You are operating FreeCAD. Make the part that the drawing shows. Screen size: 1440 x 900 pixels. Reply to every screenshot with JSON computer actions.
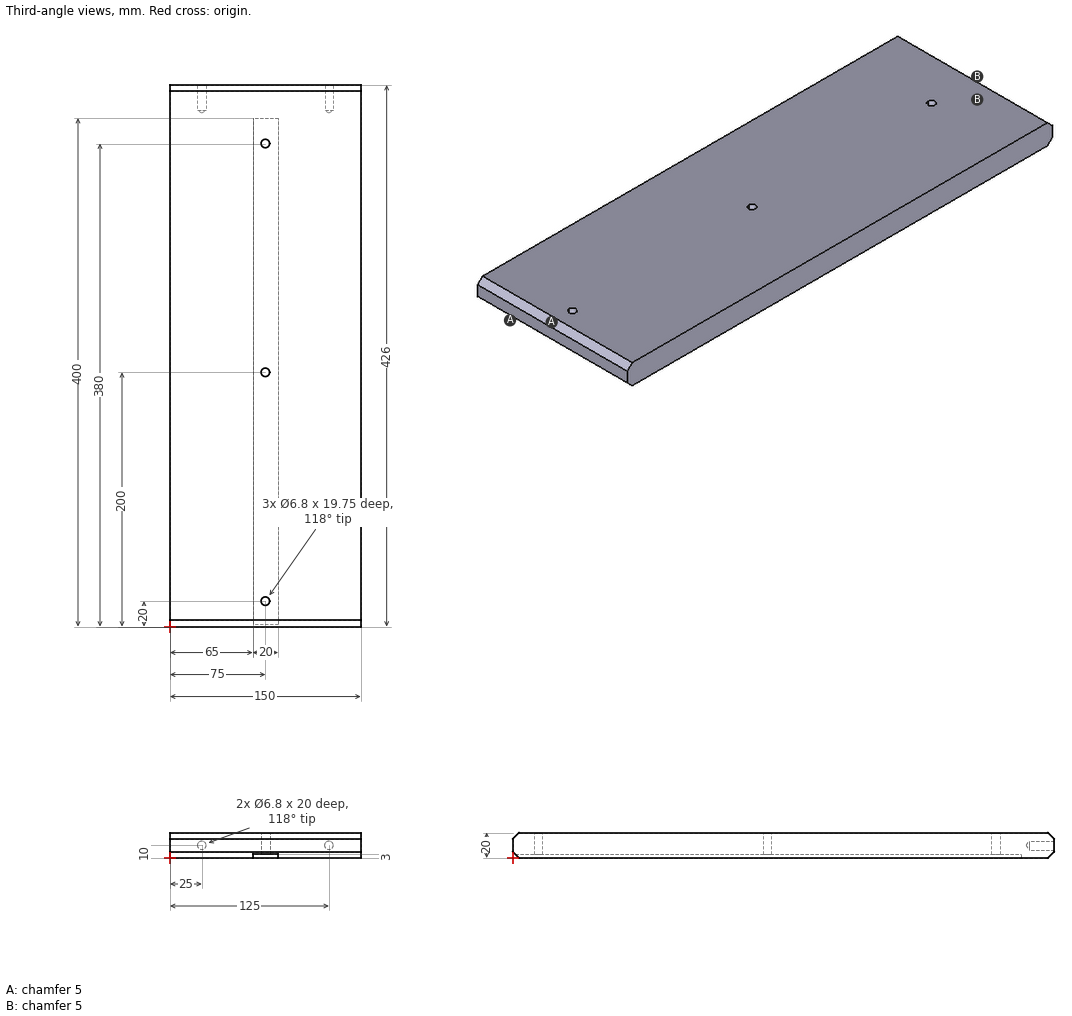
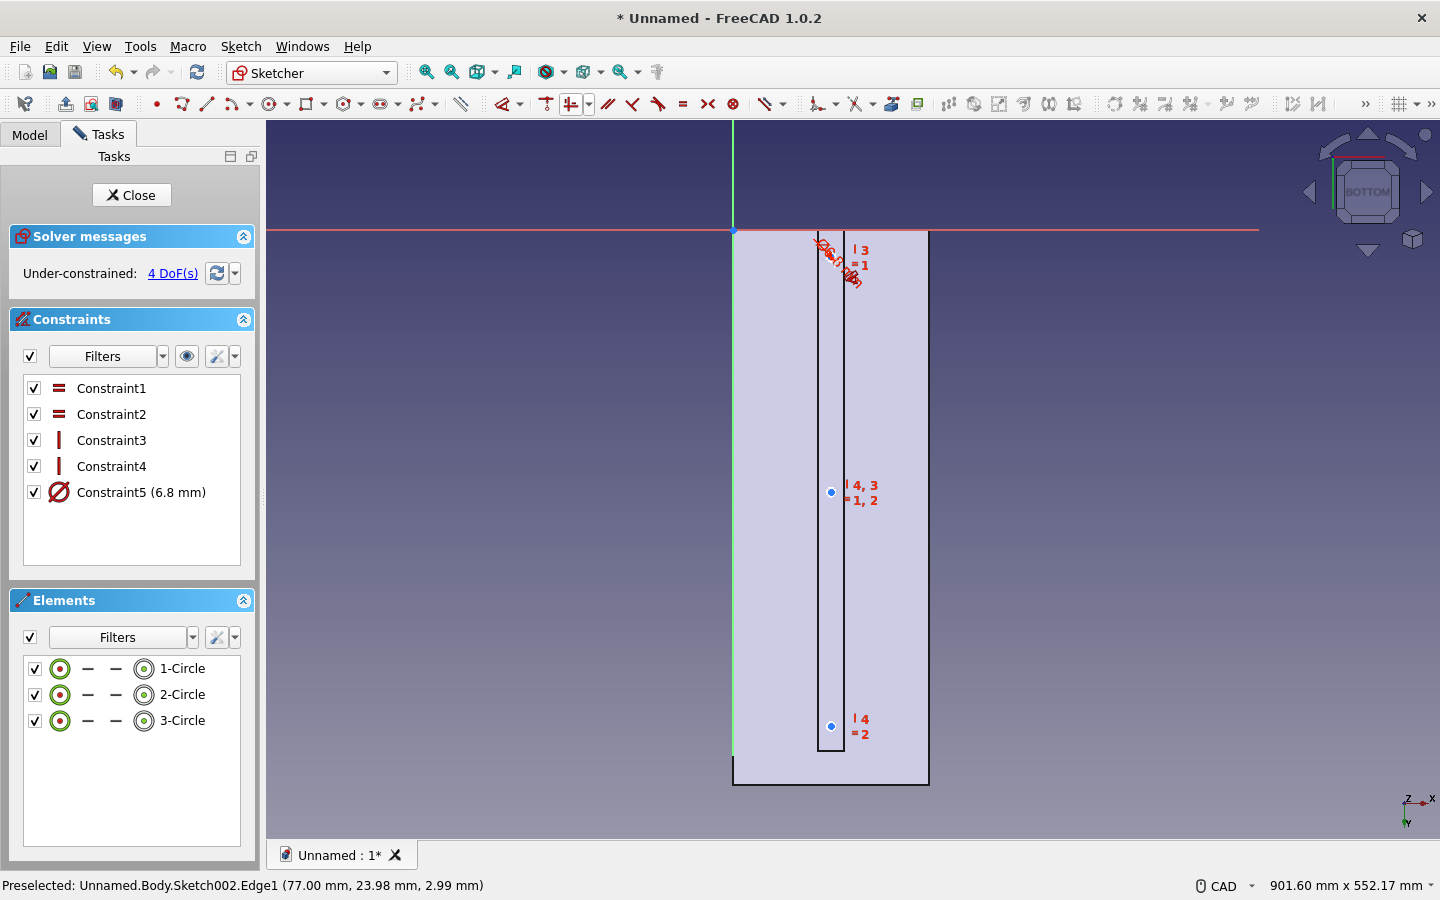
{"action": "left_click", "coordinate": [831, 257]}
{"action": "left_click", "coordinate": [782, 196]}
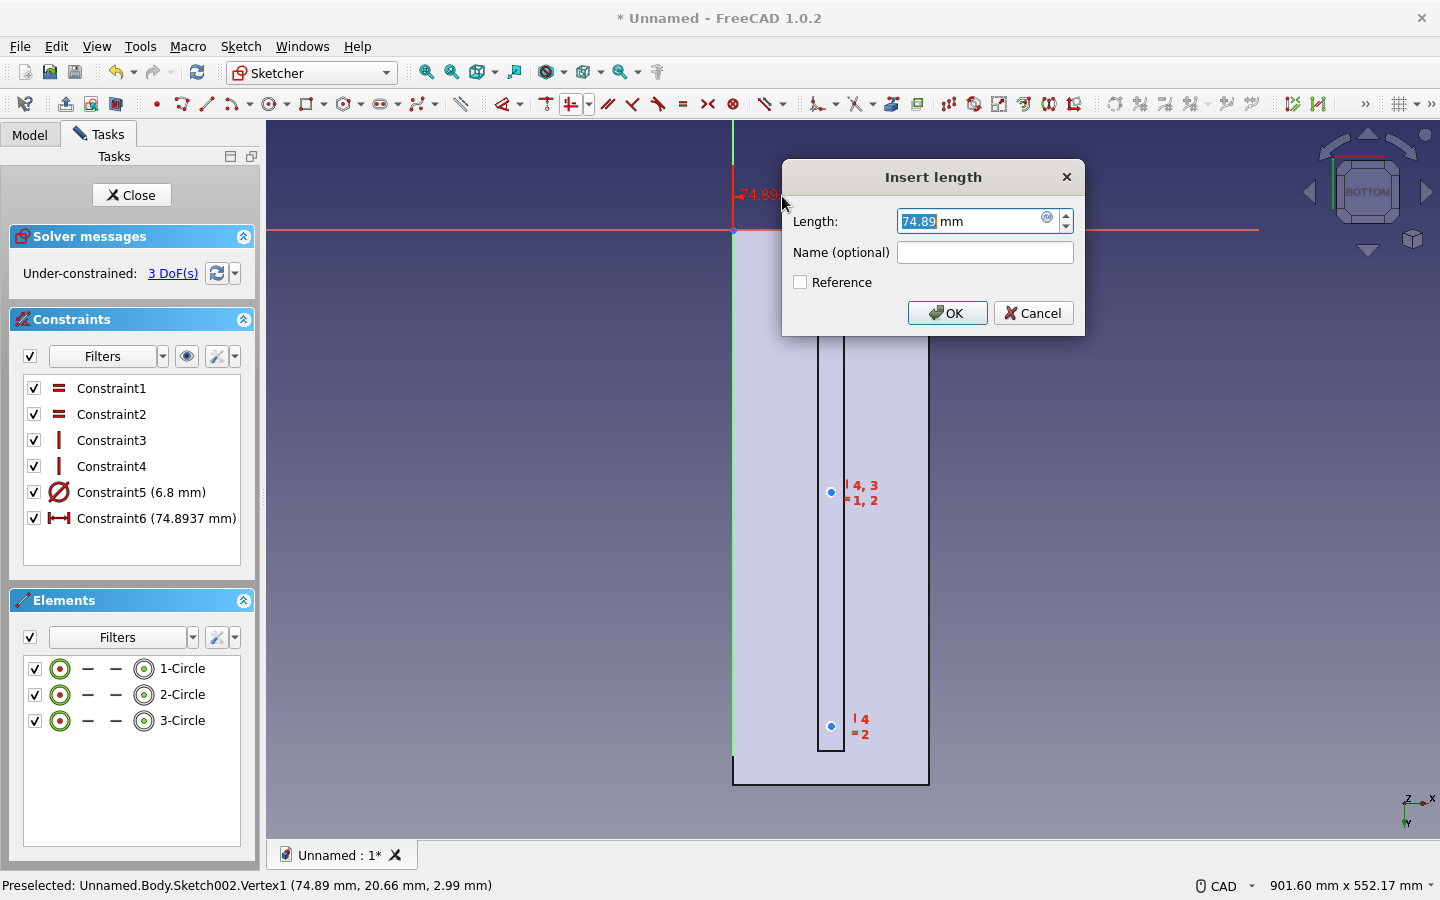
{"action": "type", "text": "75"}
{"action": "key", "text": "Return"}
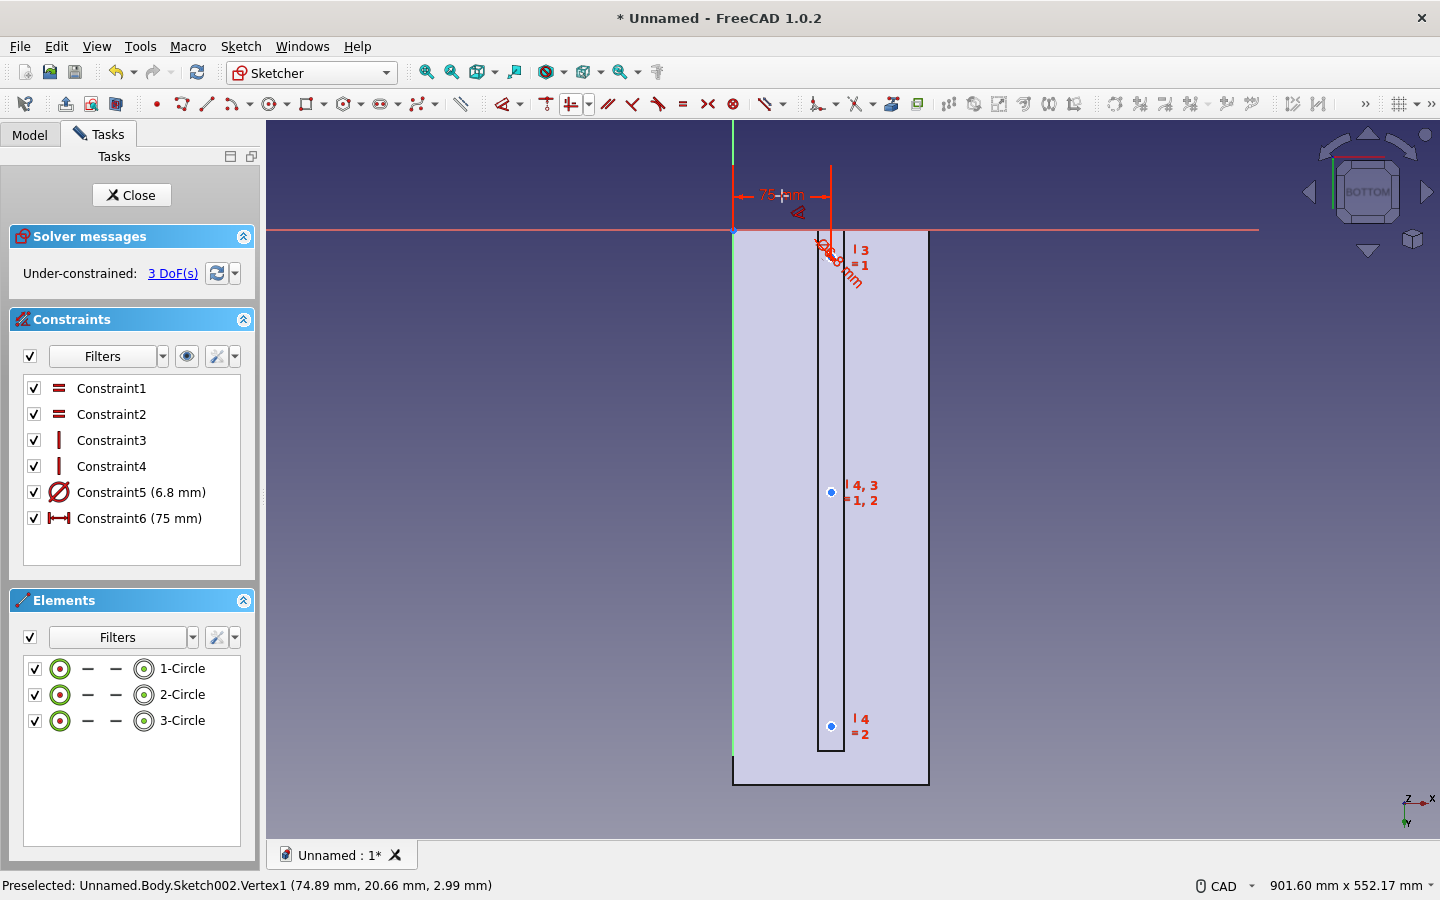
{"action": "scroll", "coordinate": [831, 257], "scroll_direction": "up", "scroll_amount": 3}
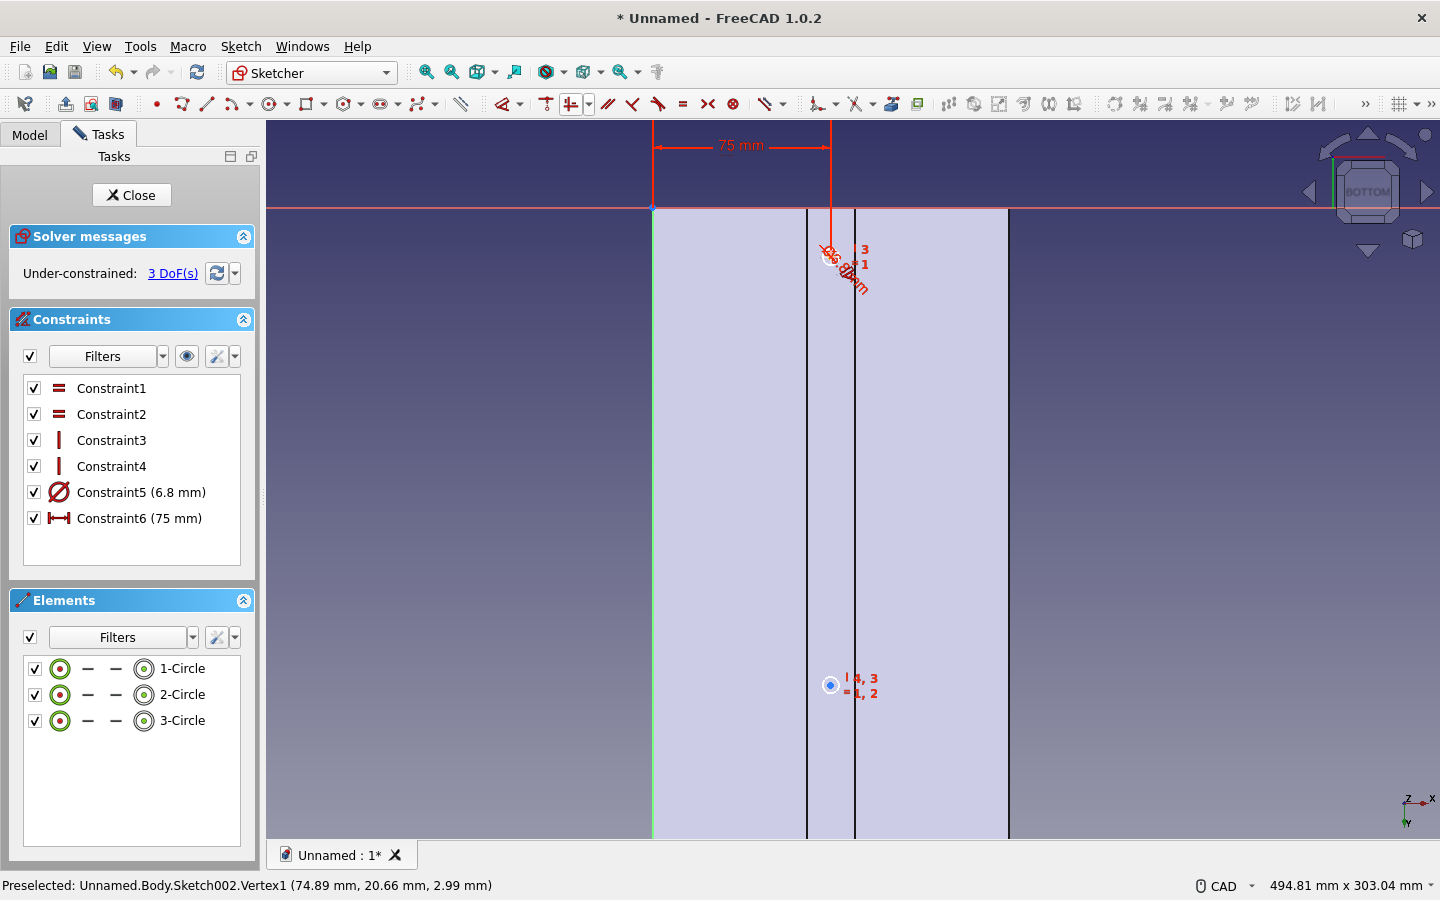
{"action": "left_click", "coordinate": [831, 257]}
{"action": "left_click", "coordinate": [619, 232]}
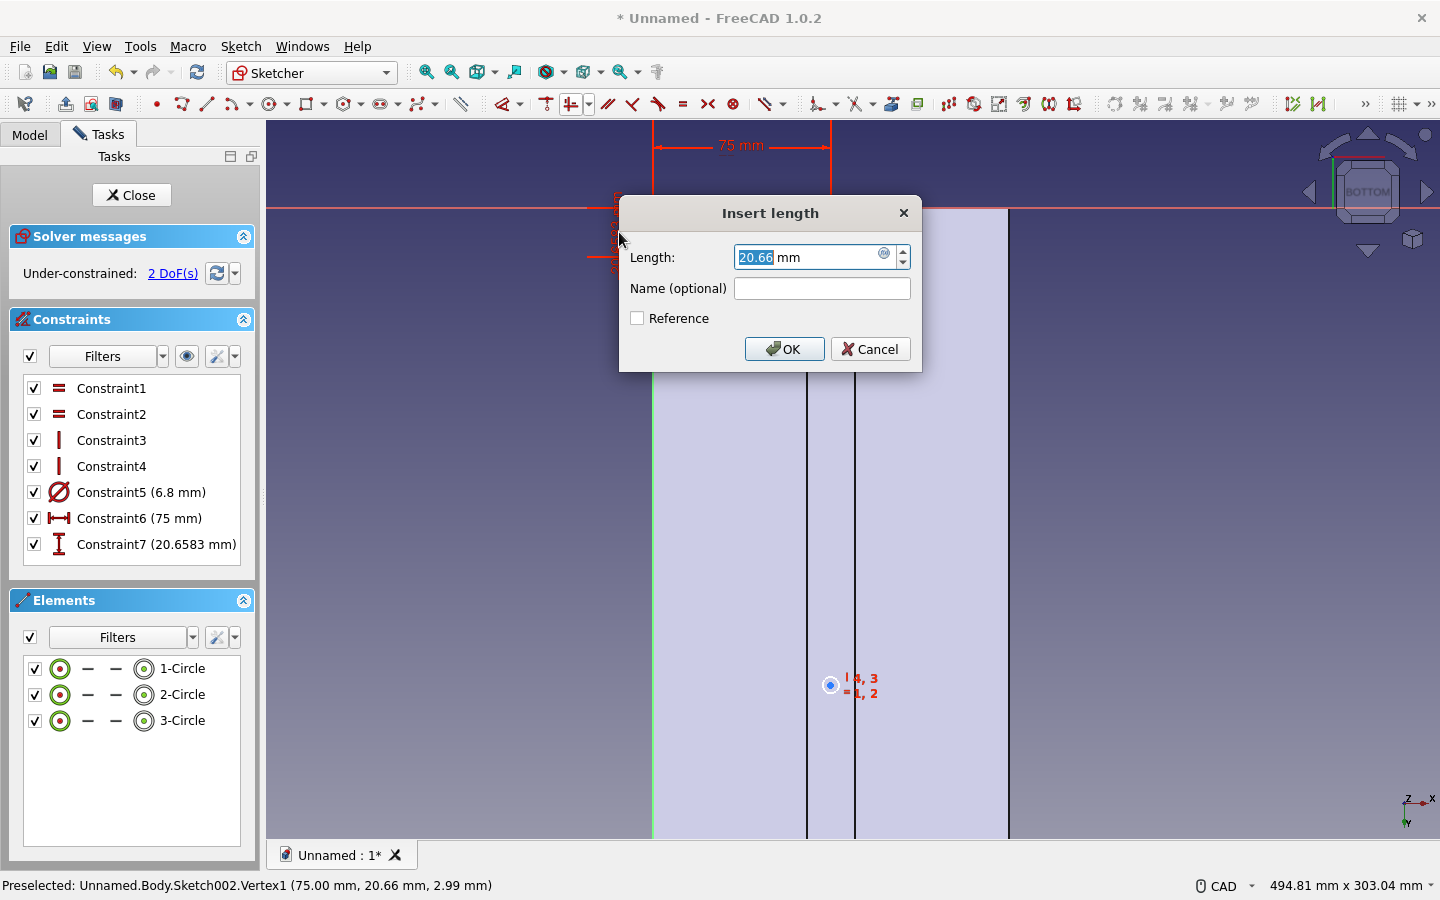
{"action": "type", "text": "20"}
{"action": "key", "text": "Return"}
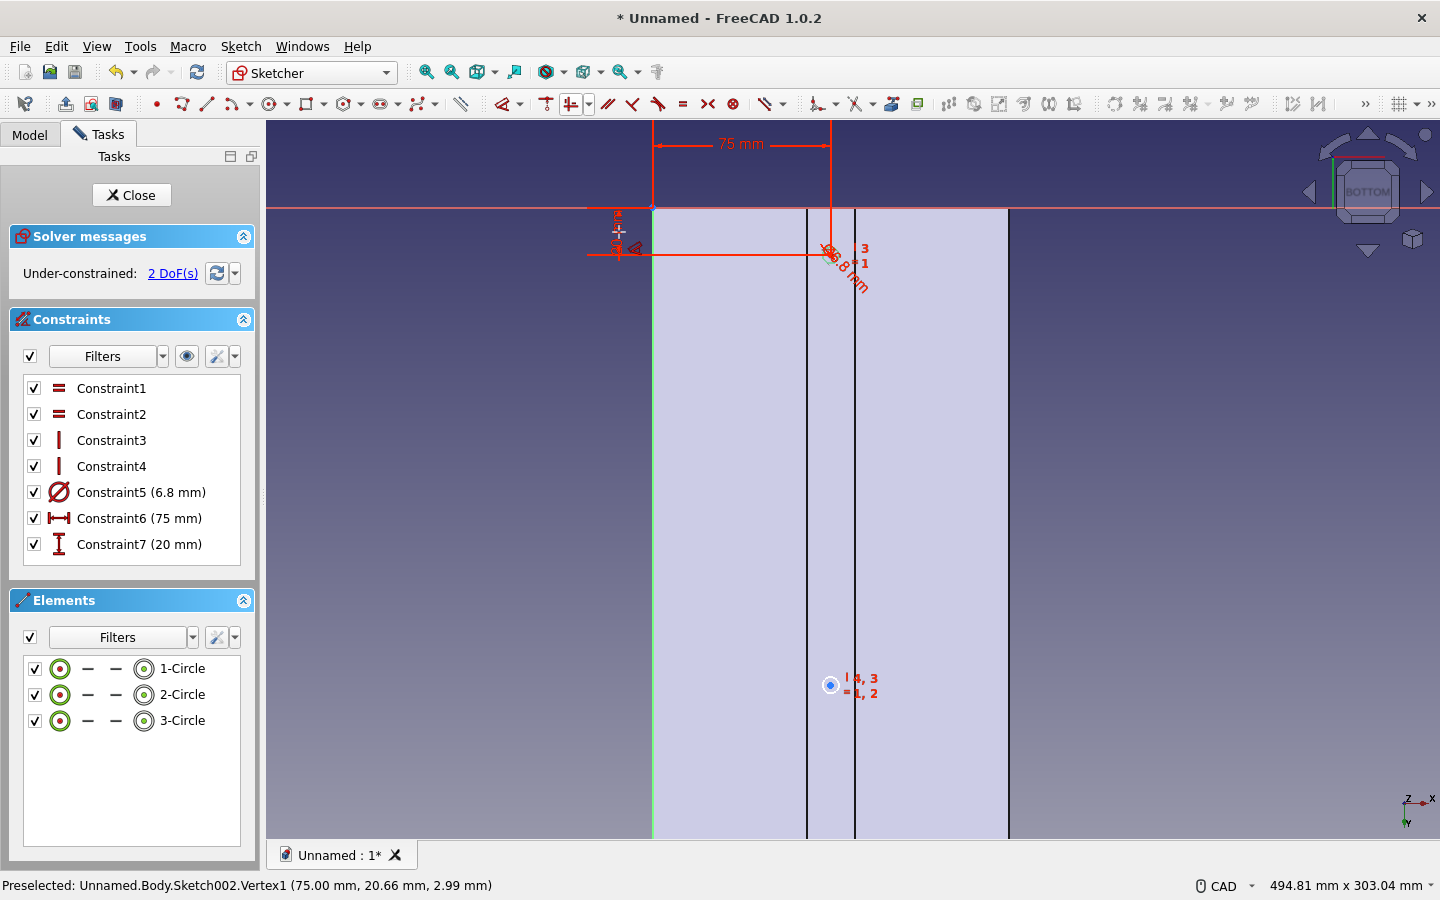
{"action": "left_click", "coordinate": [831, 685]}
{"action": "left_click", "coordinate": [619, 447]}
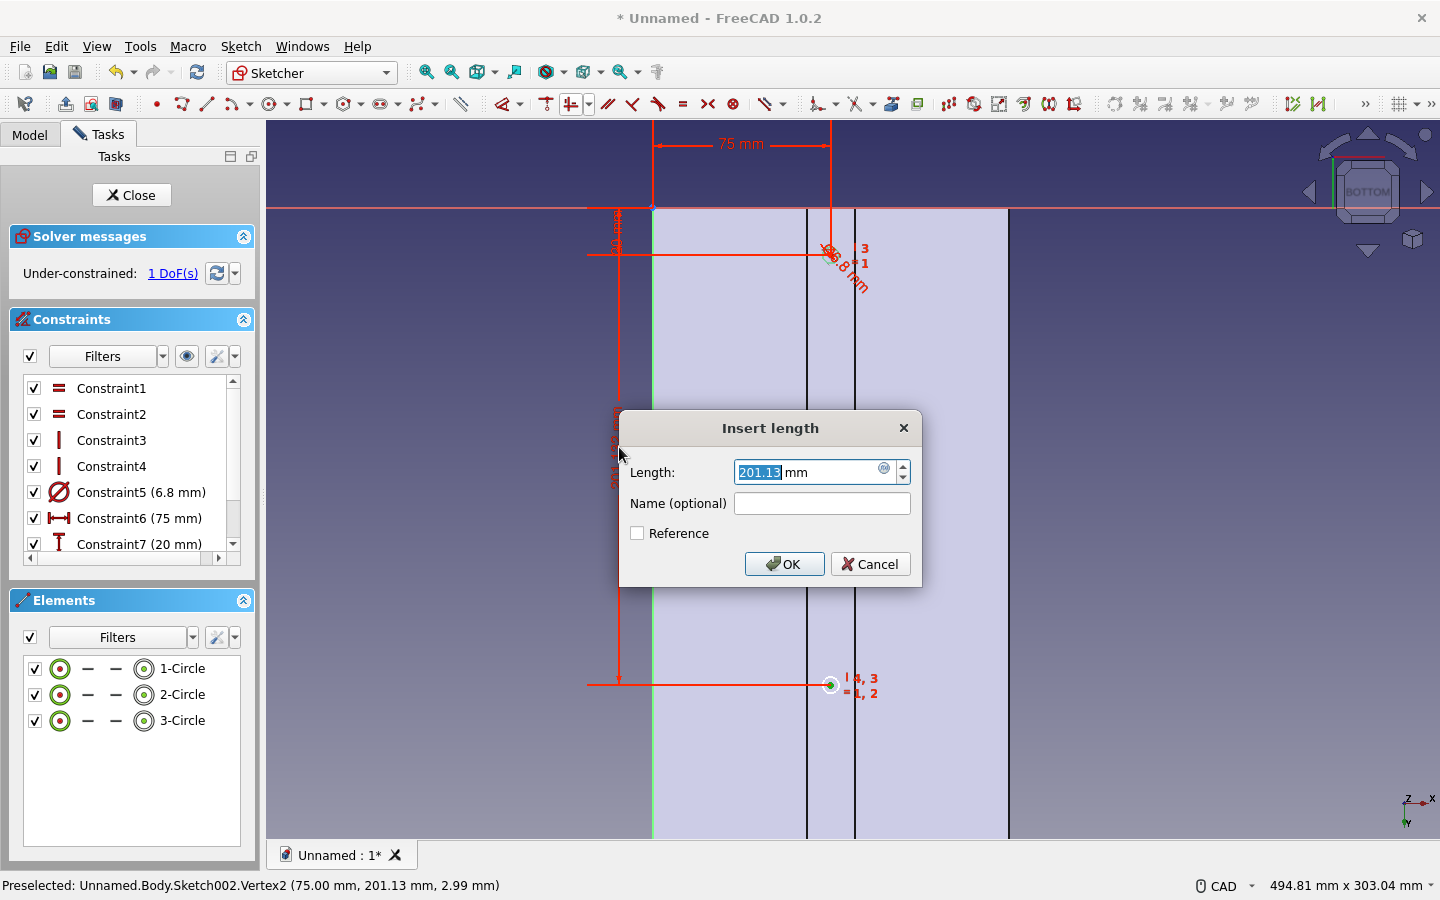
{"action": "type", "text": "200"}
{"action": "key", "text": "Return"}